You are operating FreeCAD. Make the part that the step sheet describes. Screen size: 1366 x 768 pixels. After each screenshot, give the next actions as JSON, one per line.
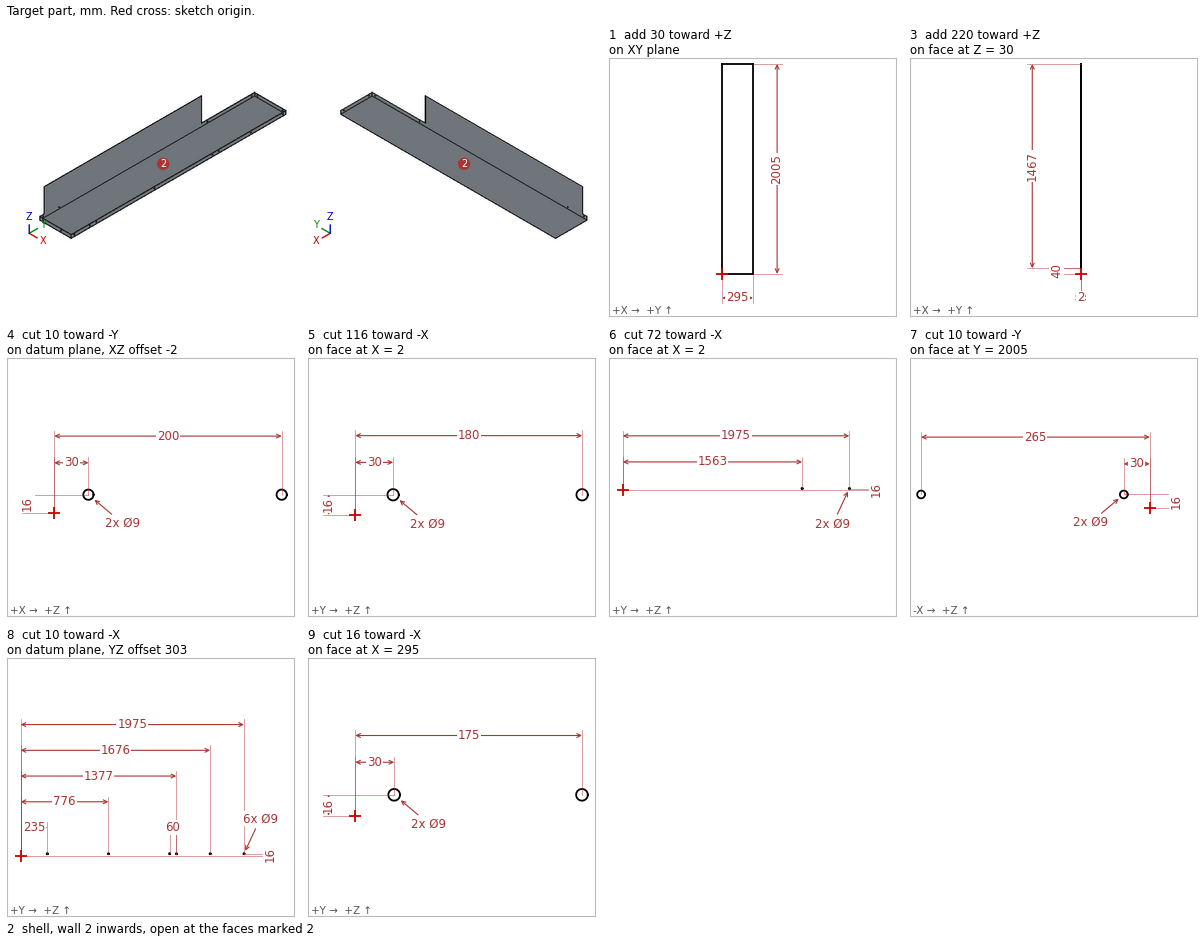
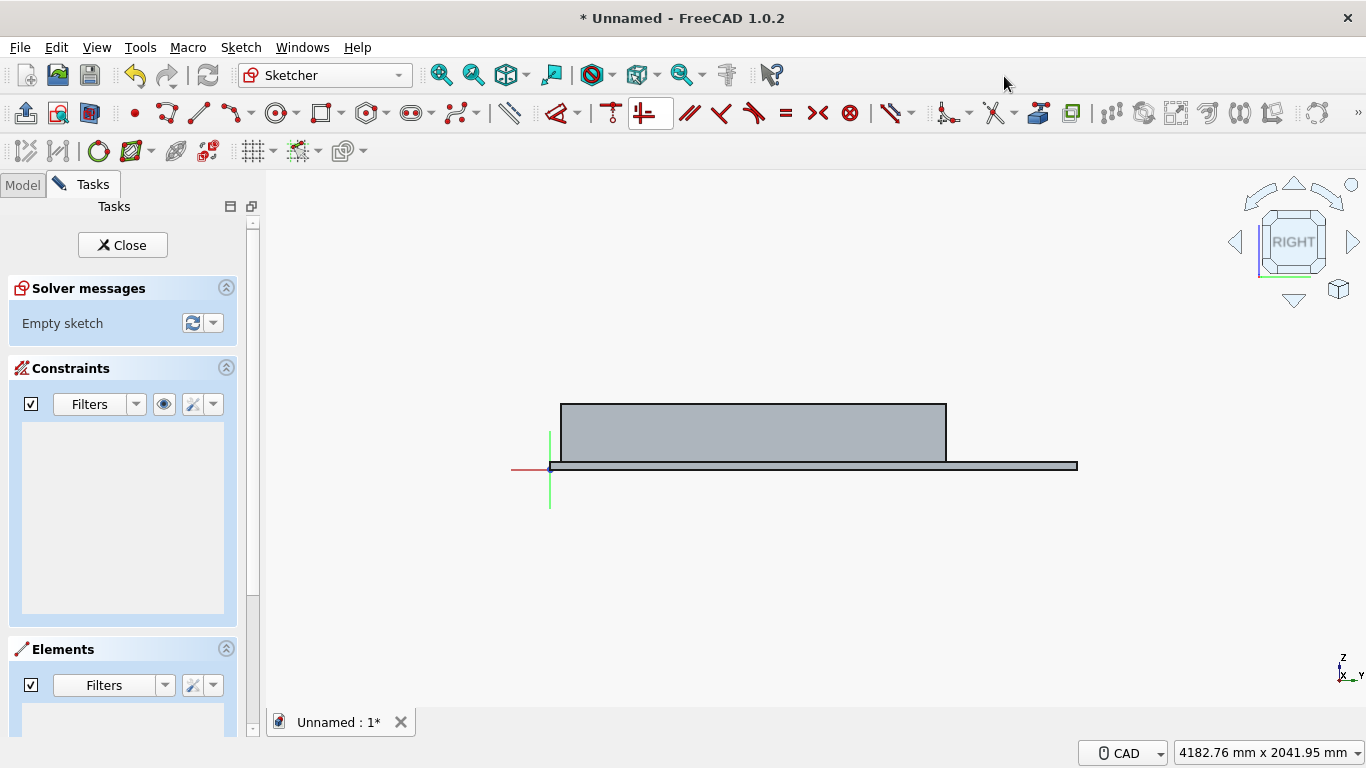
{"action": "left_click", "coordinate": [90, 114]}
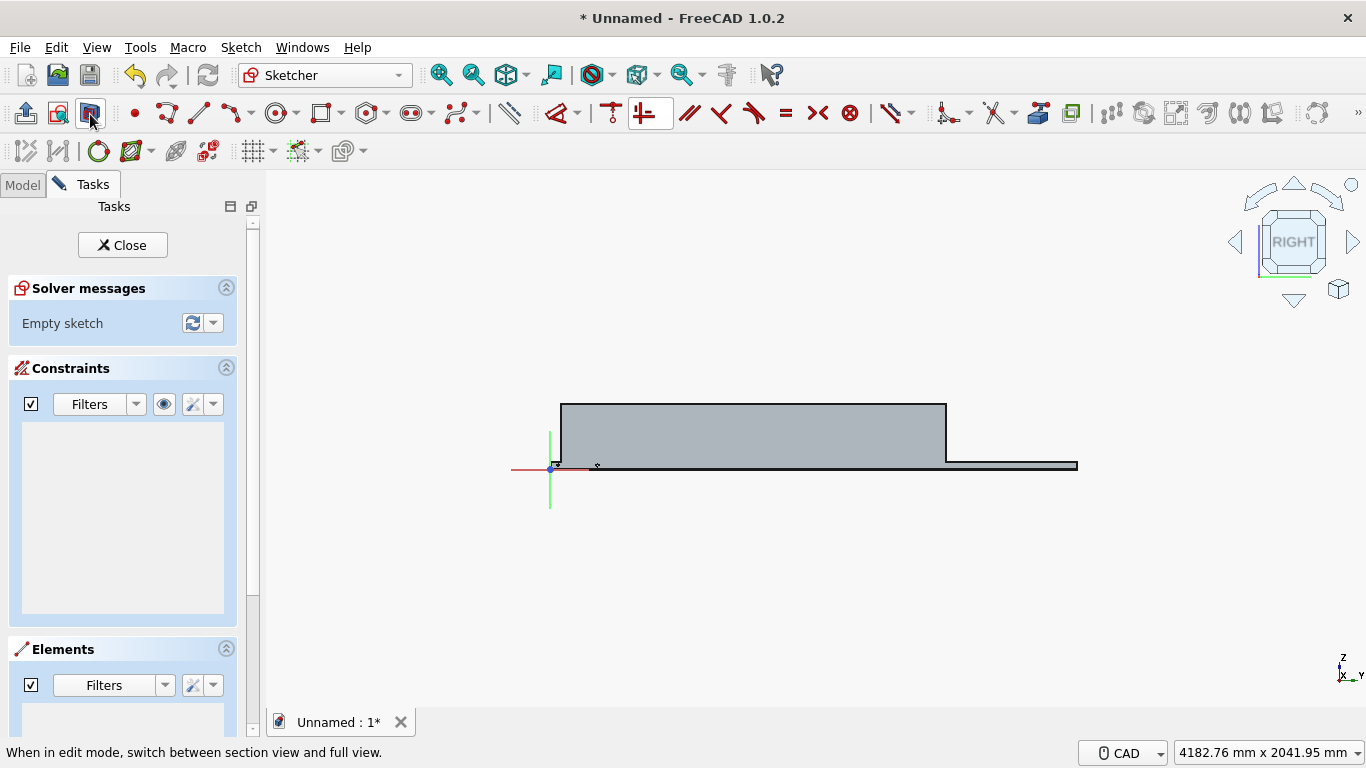
{"action": "scroll", "coordinate": [1068, 471], "scroll_direction": "up", "scroll_amount": 9}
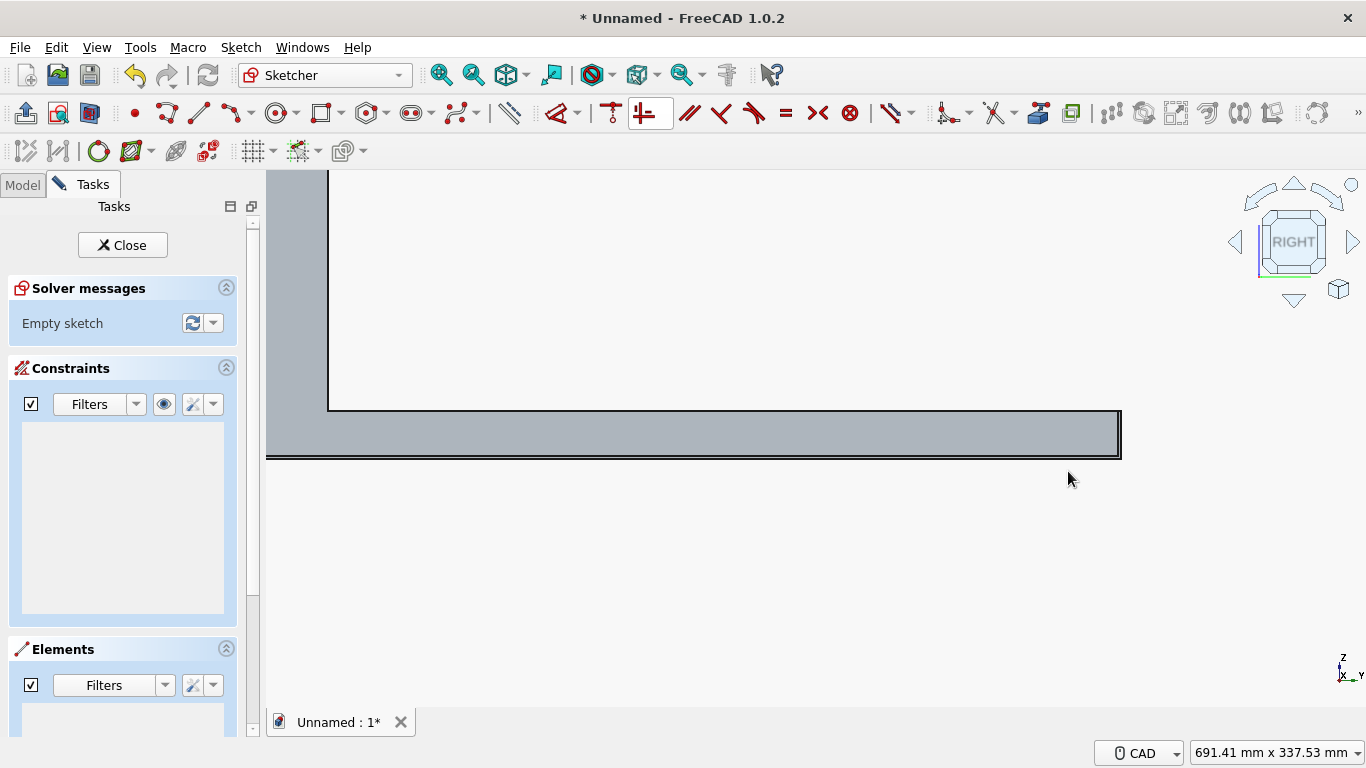
{"action": "left_click", "coordinate": [276, 114]}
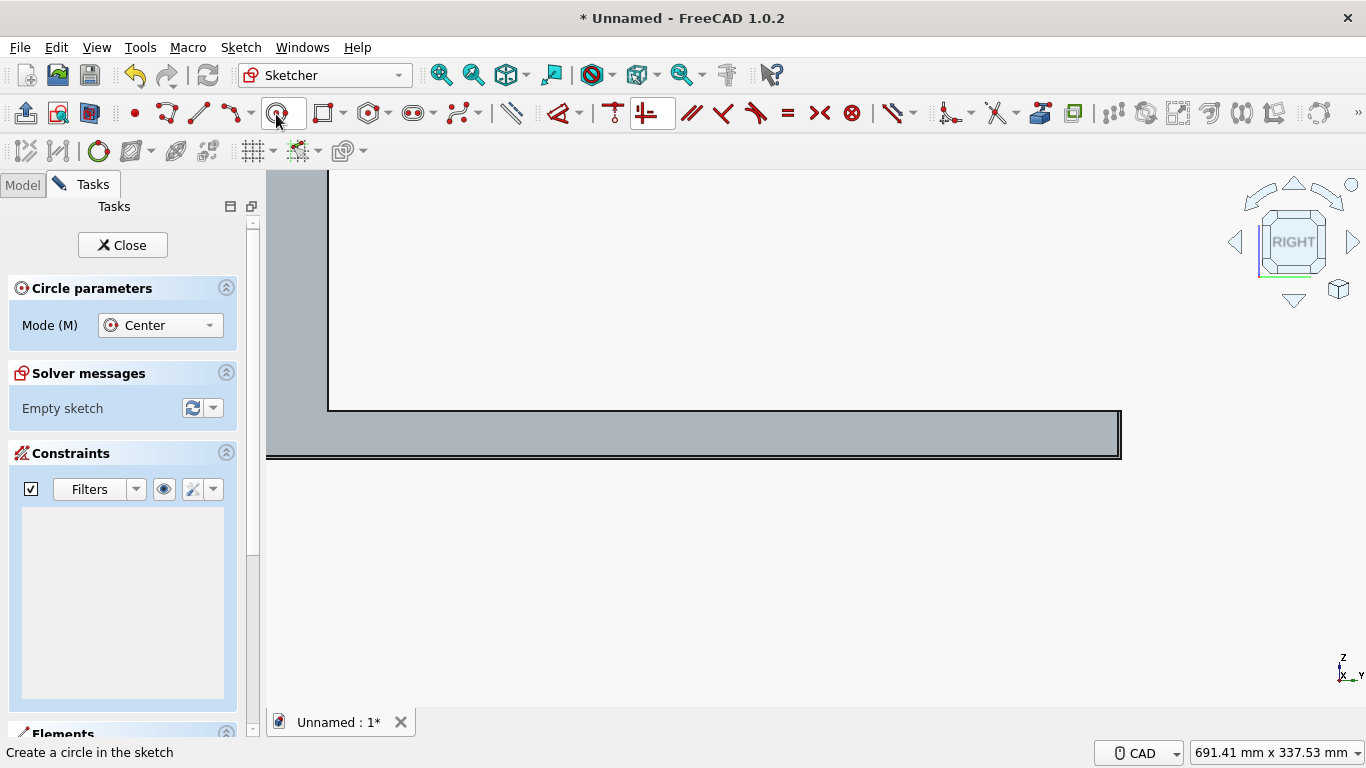
{"action": "scroll", "coordinate": [1073, 434], "scroll_direction": "up", "scroll_amount": 6}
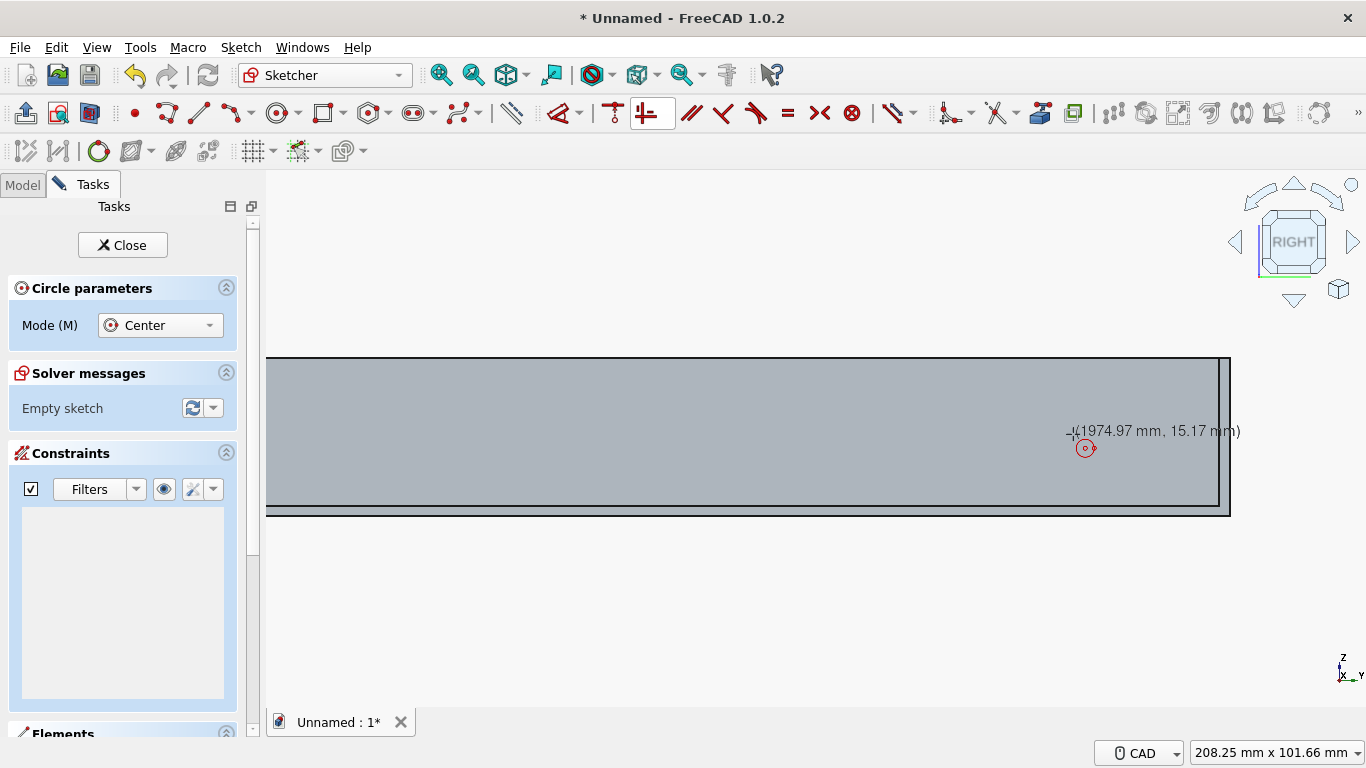
{"action": "left_click", "coordinate": [1071, 432]}
{"action": "left_click", "coordinate": [1088, 415]}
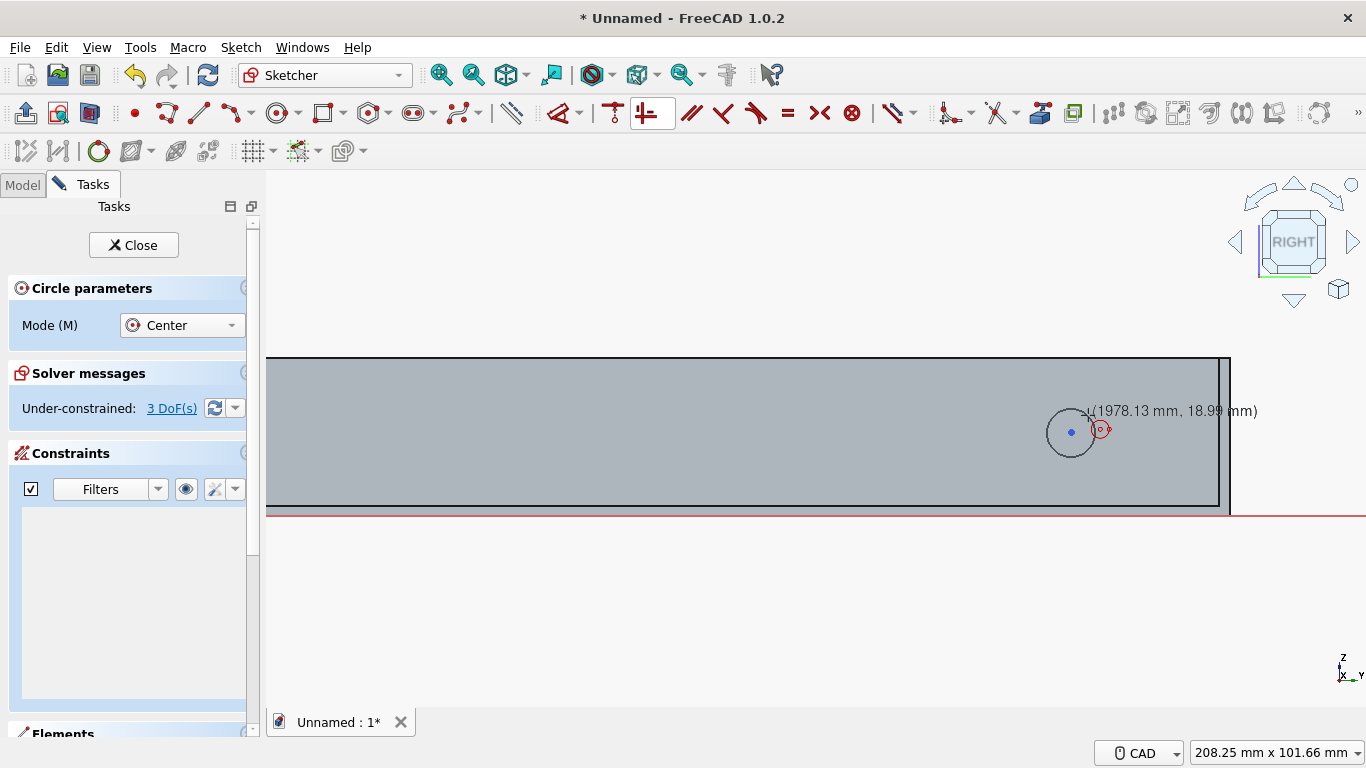
{"action": "scroll", "coordinate": [1077, 441], "scroll_direction": "down", "scroll_amount": 6}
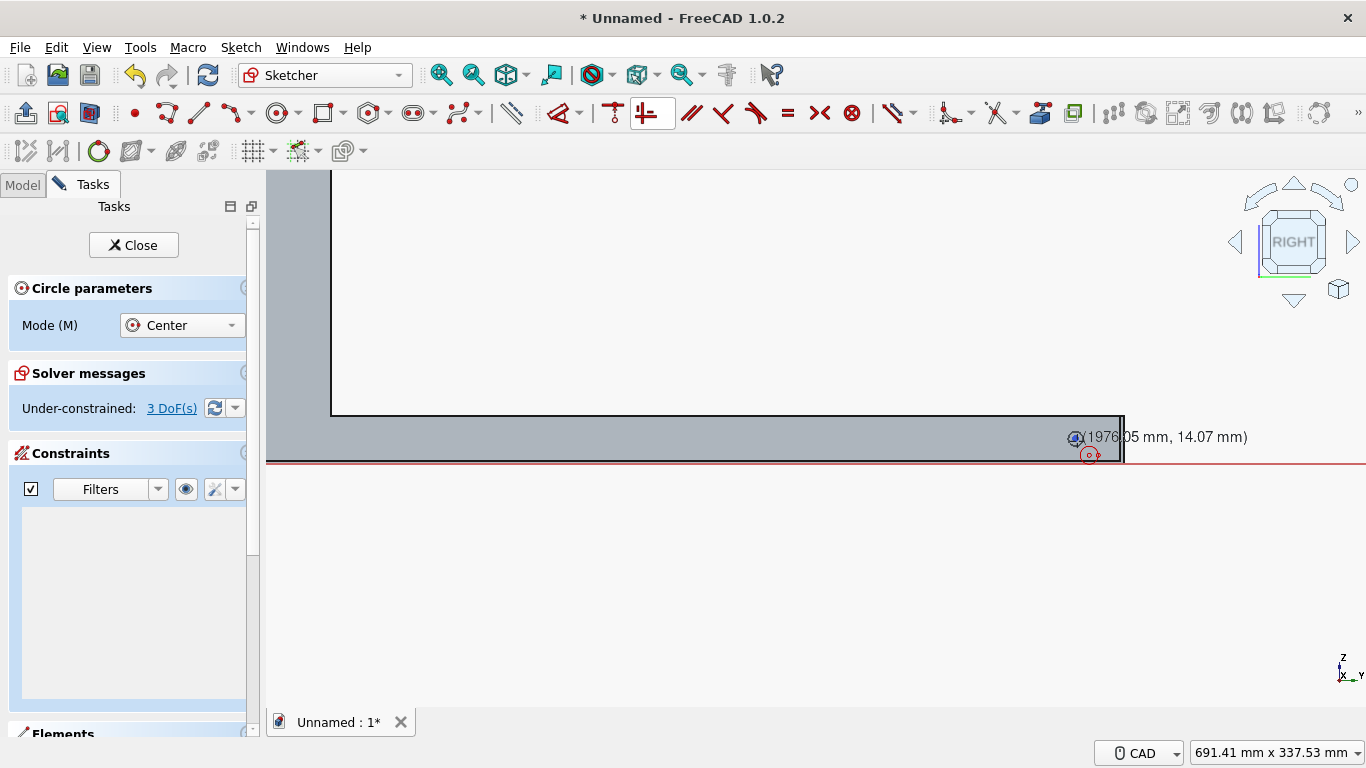
{"action": "scroll", "coordinate": [420, 439], "scroll_direction": "up", "scroll_amount": 6}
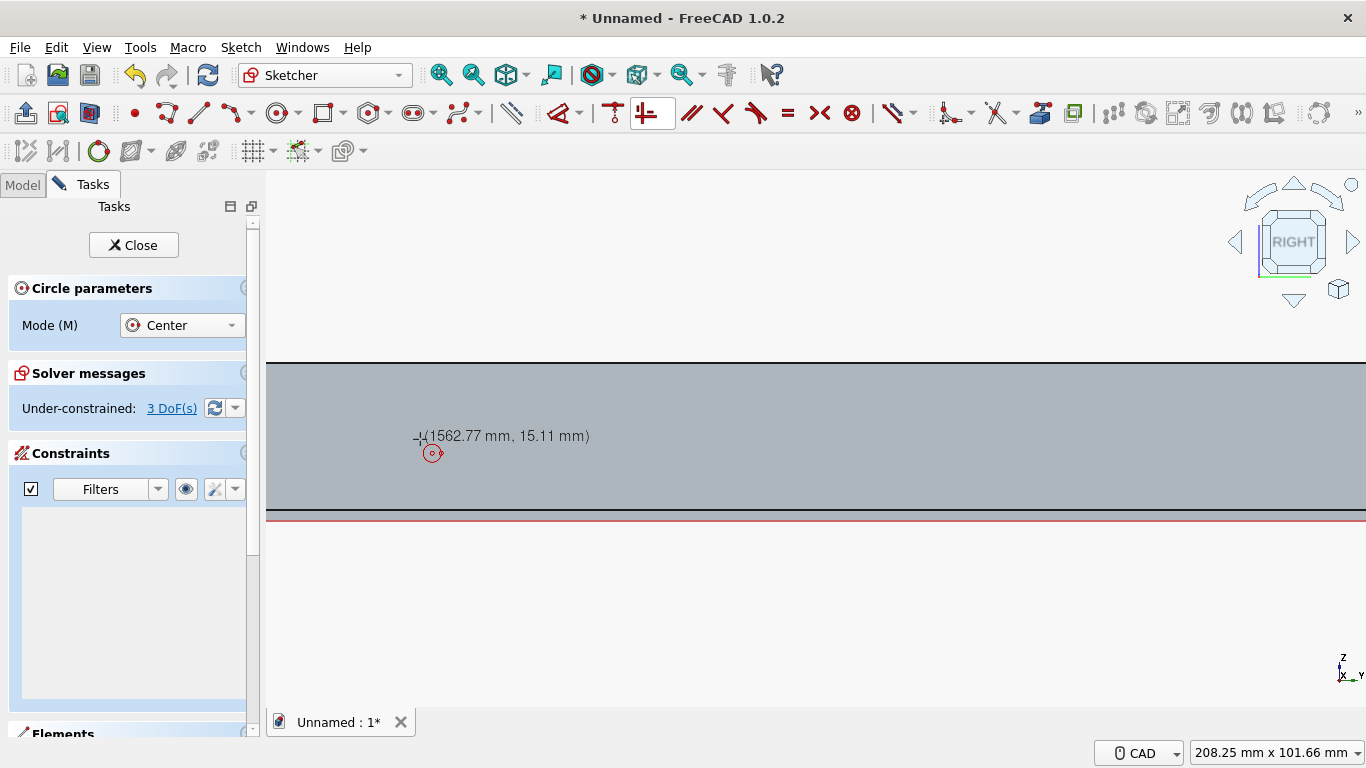
{"action": "left_click", "coordinate": [421, 436]}
{"action": "left_click", "coordinate": [438, 420]}
{"action": "key", "text": "Escape"}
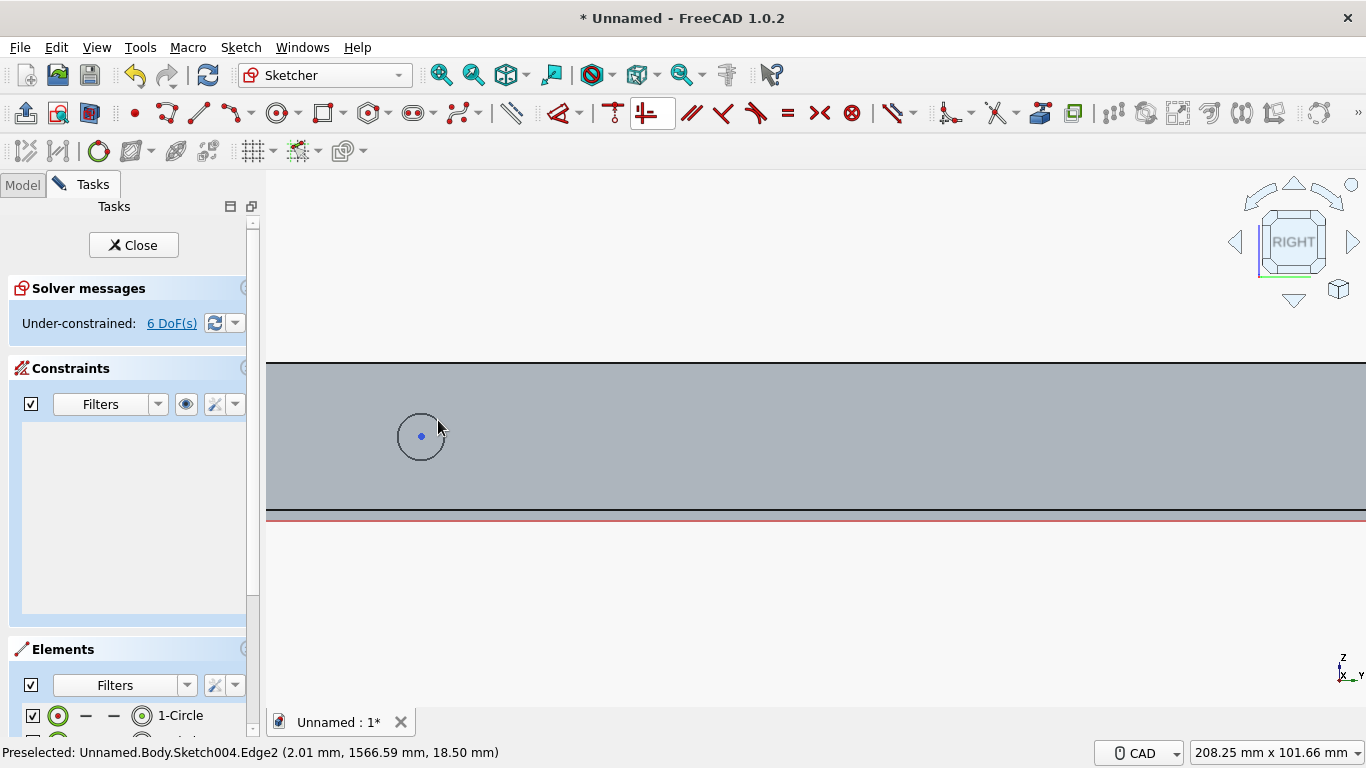
{"action": "scroll", "coordinate": [419, 439], "scroll_direction": "down", "scroll_amount": 6}